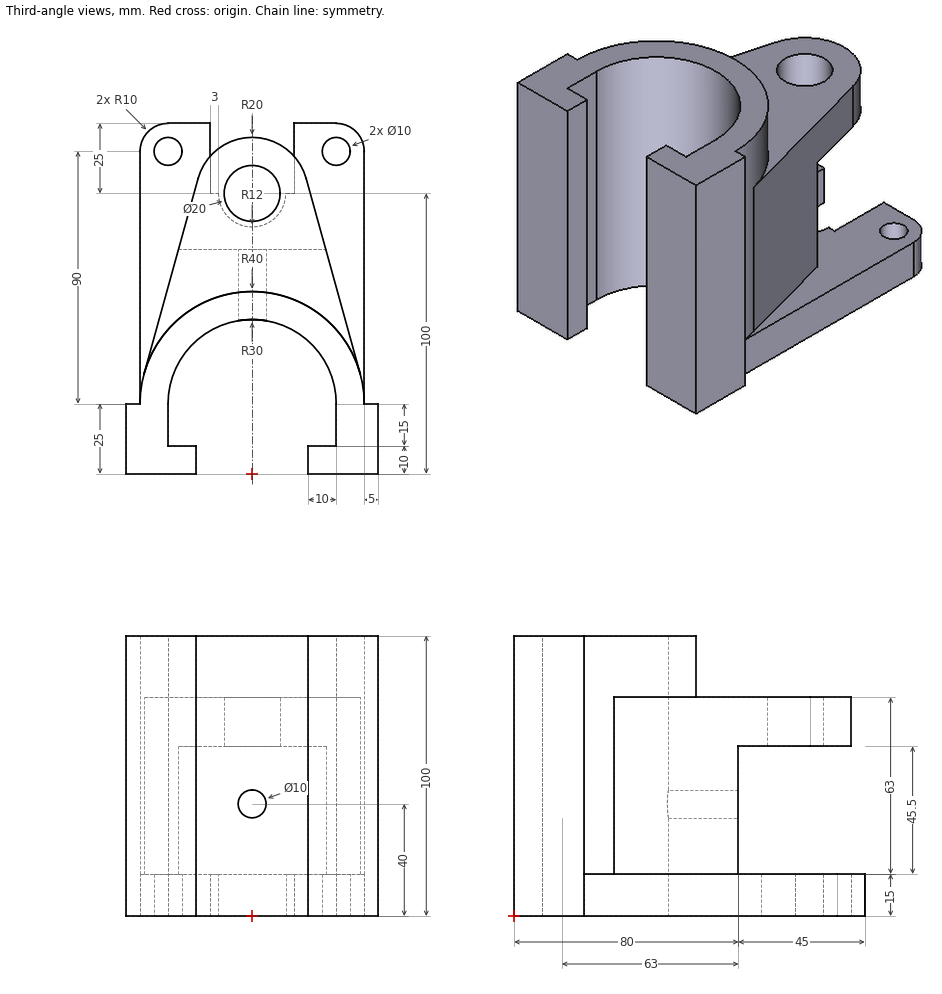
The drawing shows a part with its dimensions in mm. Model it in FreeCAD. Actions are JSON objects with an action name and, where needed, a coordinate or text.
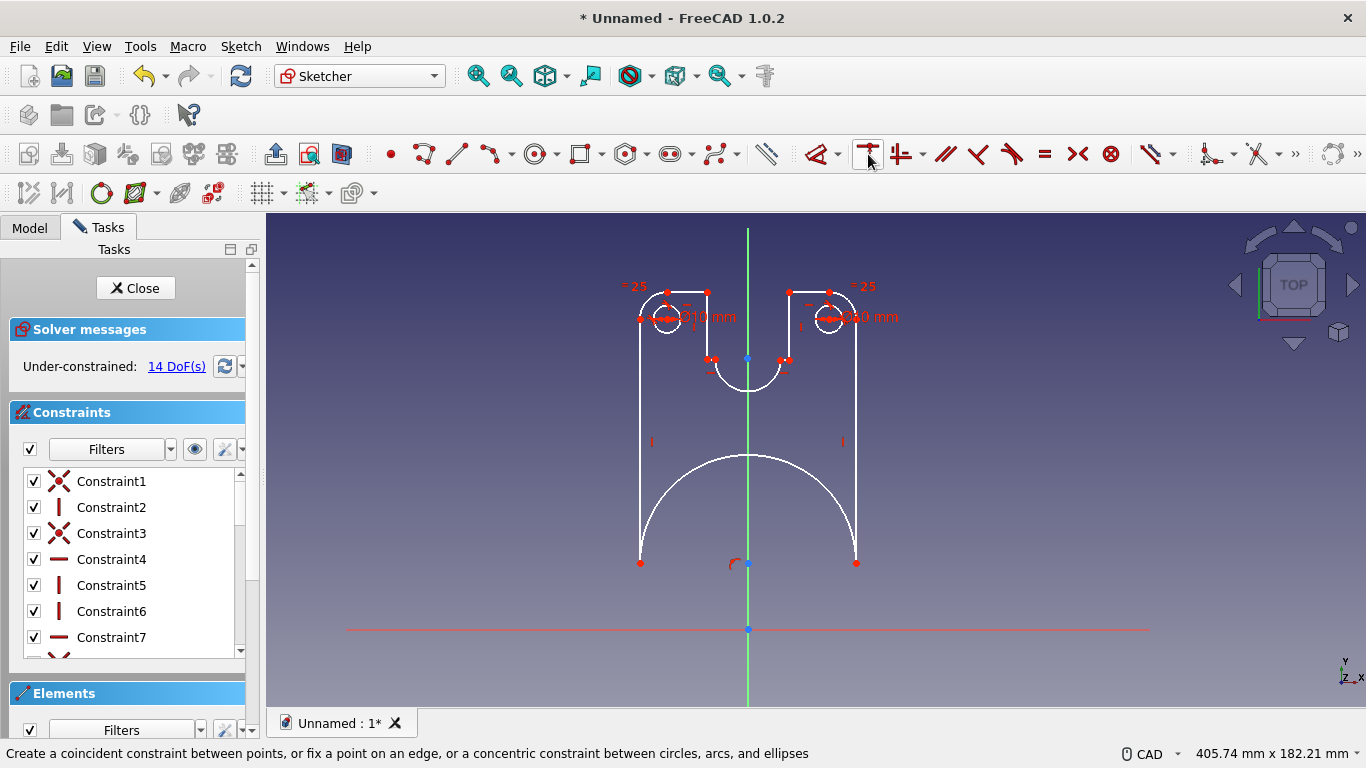
{"action": "left_click", "coordinate": [748, 359]}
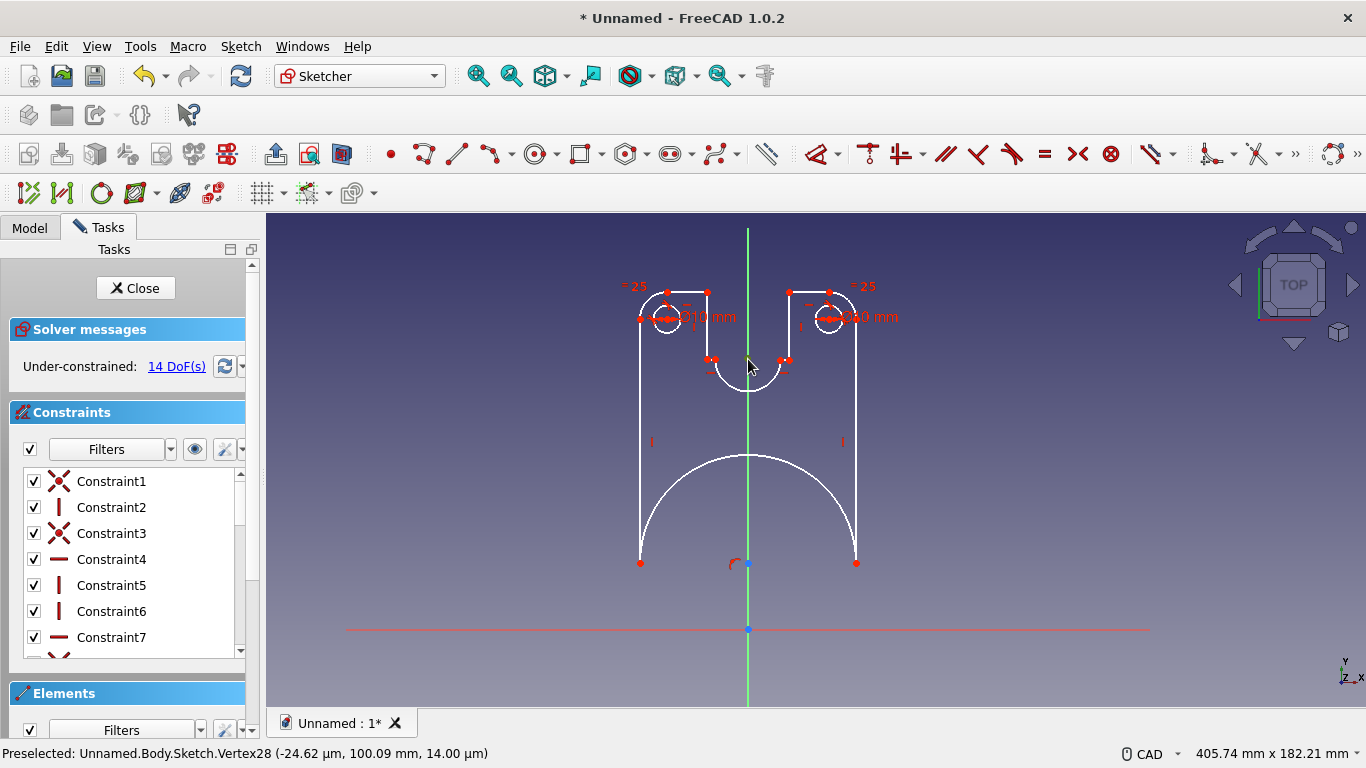
{"action": "left_click", "coordinate": [748, 585]}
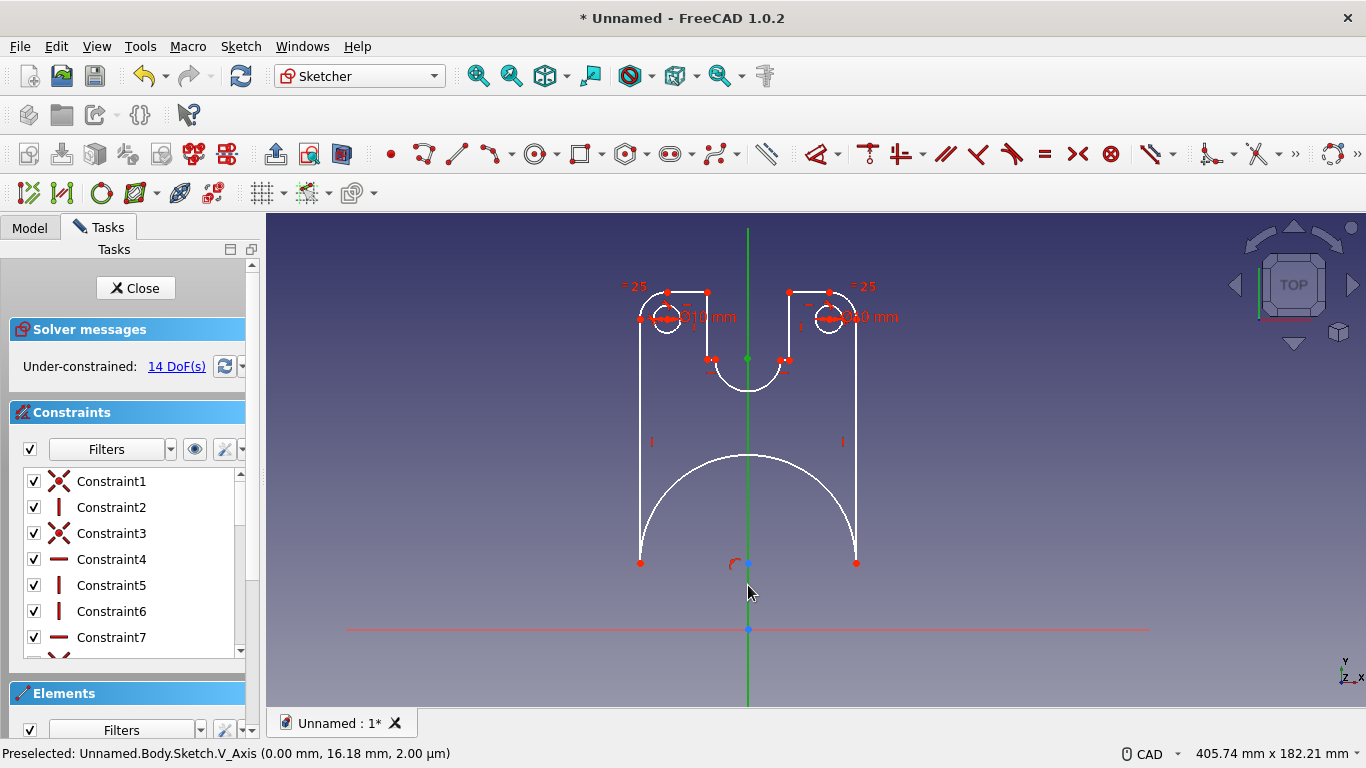
{"action": "left_click", "coordinate": [868, 154]}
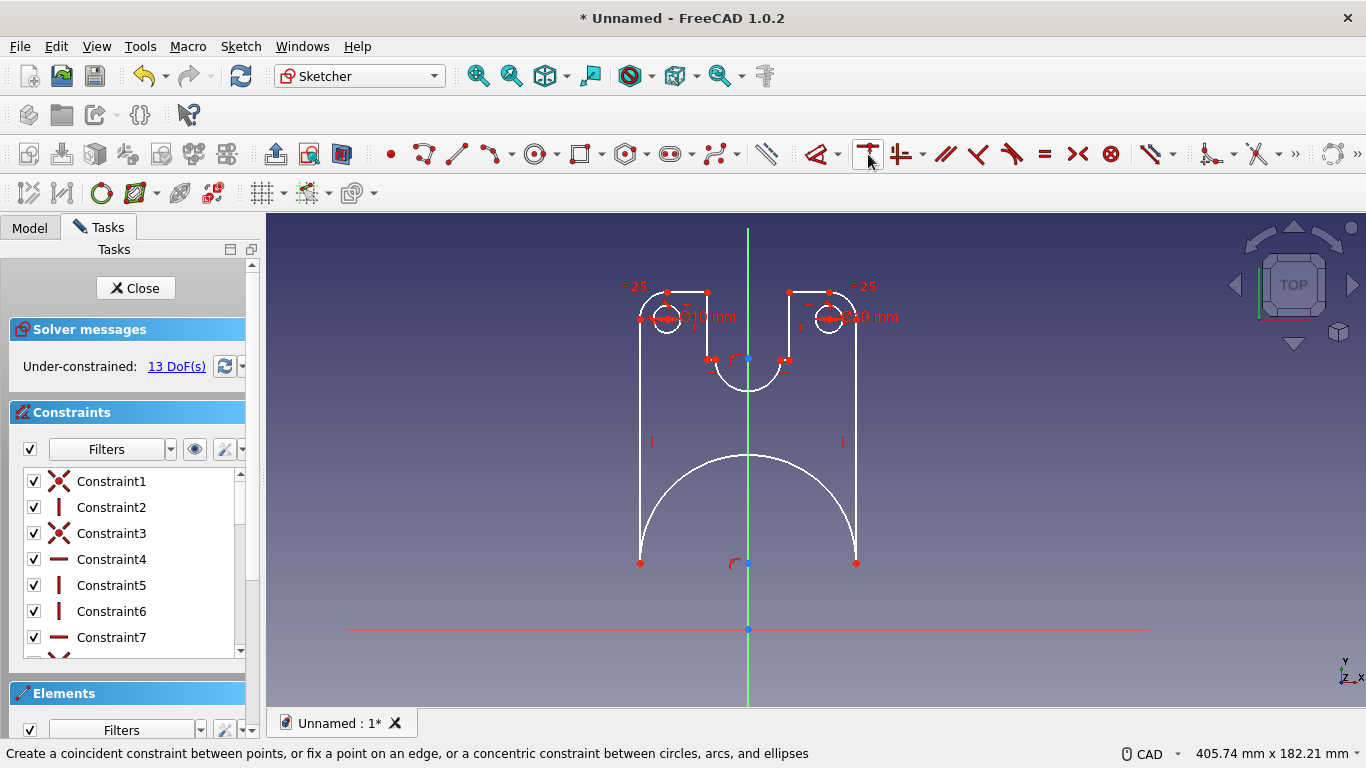
{"action": "left_click", "coordinate": [707, 292]}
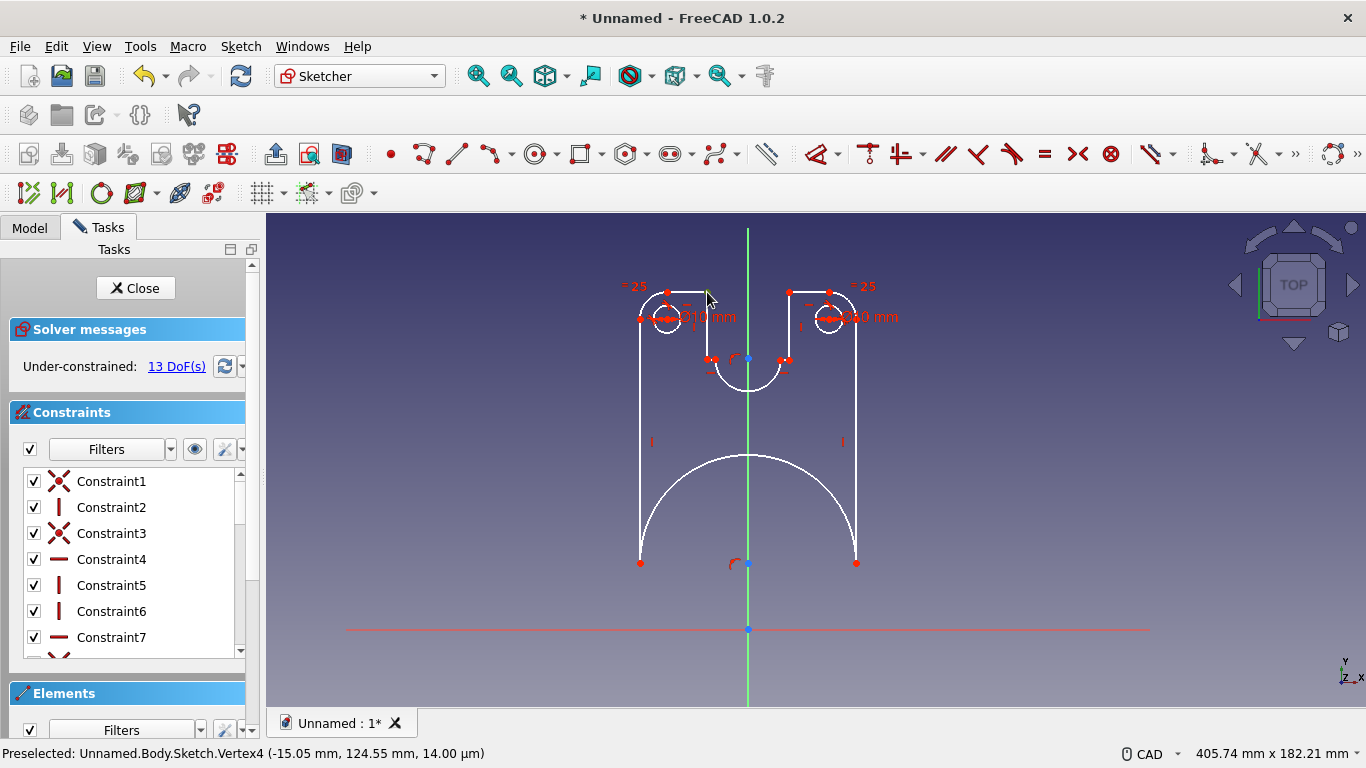
{"action": "left_click", "coordinate": [789, 292]}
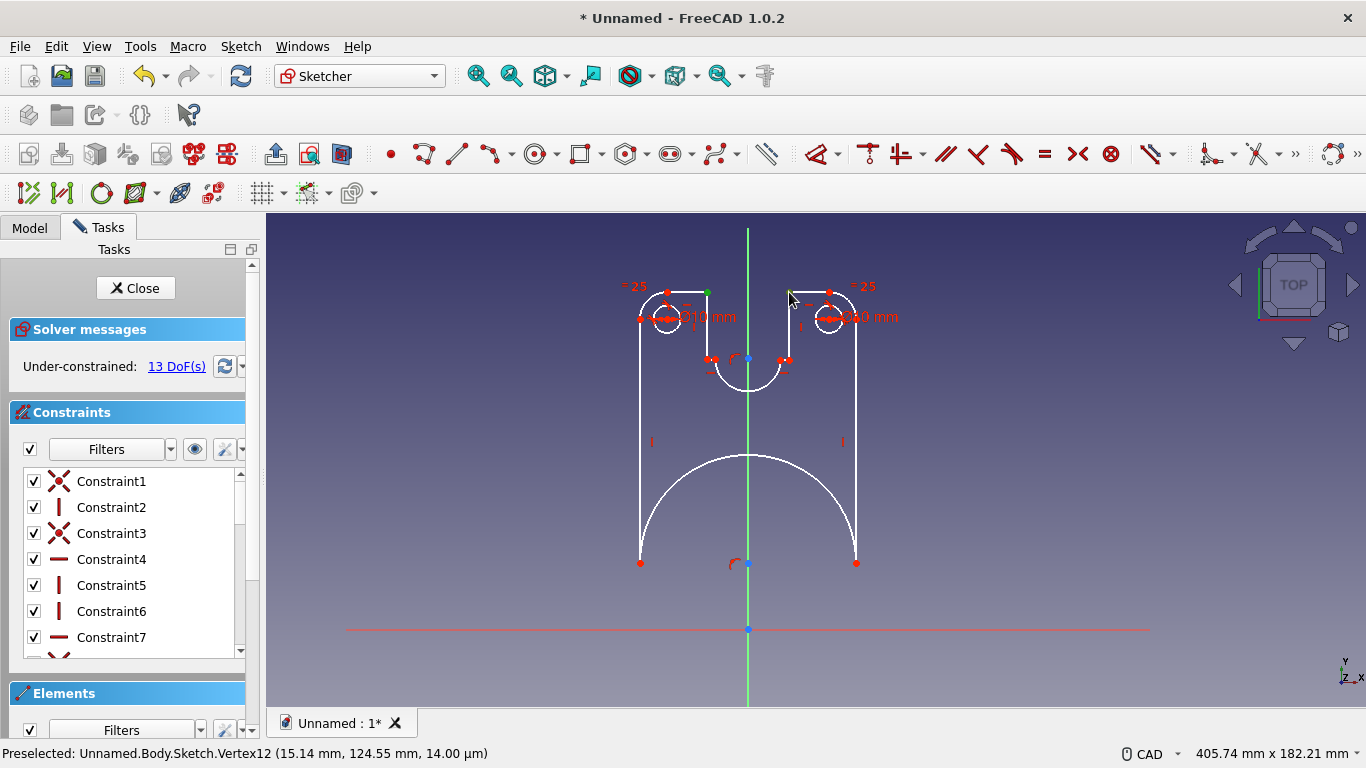
{"action": "left_click", "coordinate": [748, 585]}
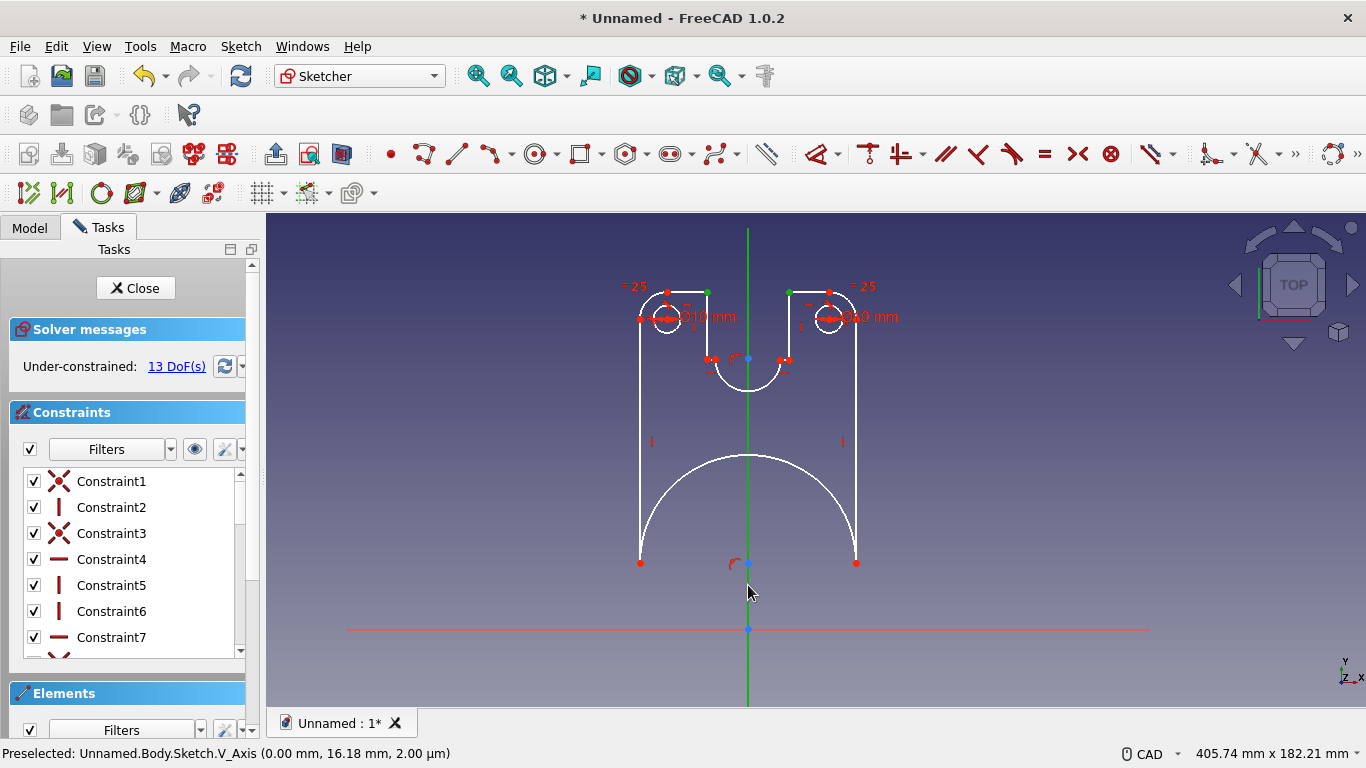
{"action": "left_click", "coordinate": [1078, 154]}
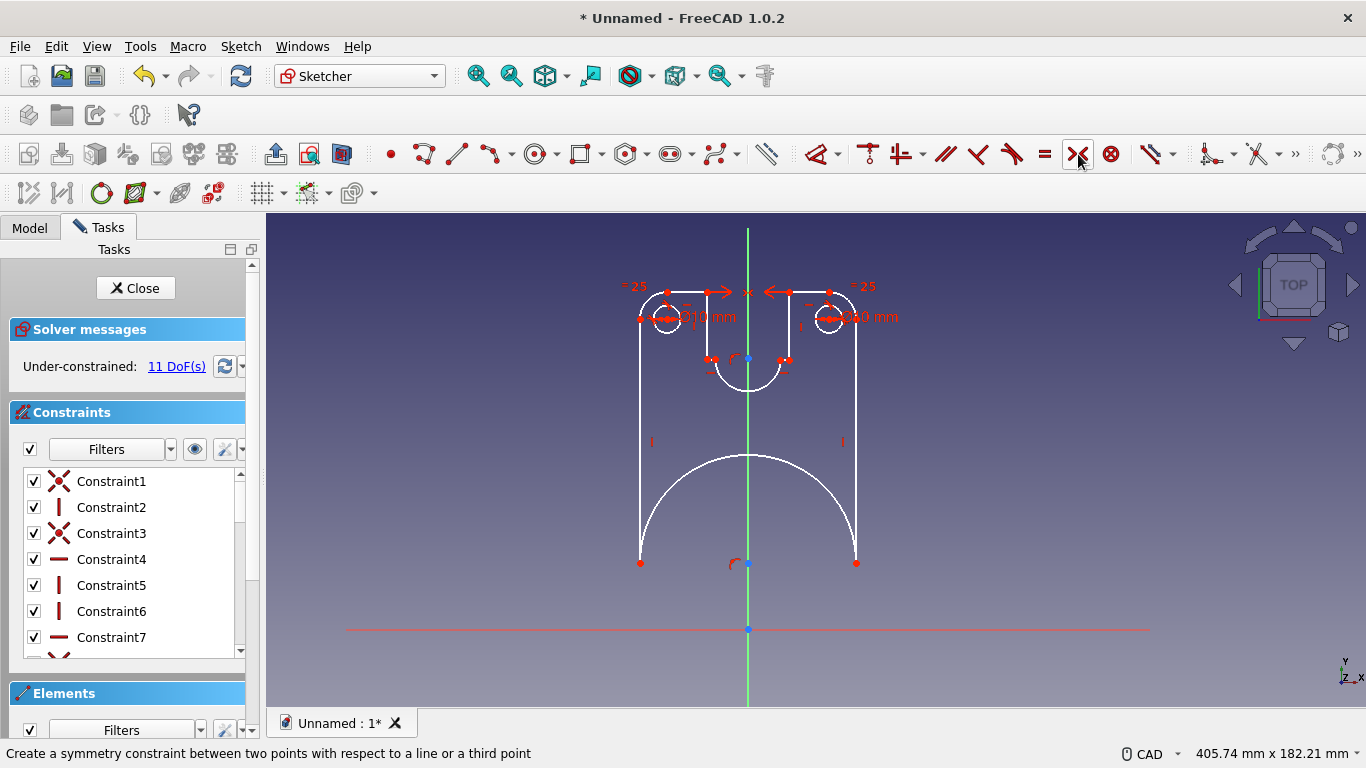
{"action": "left_click", "coordinate": [816, 154]}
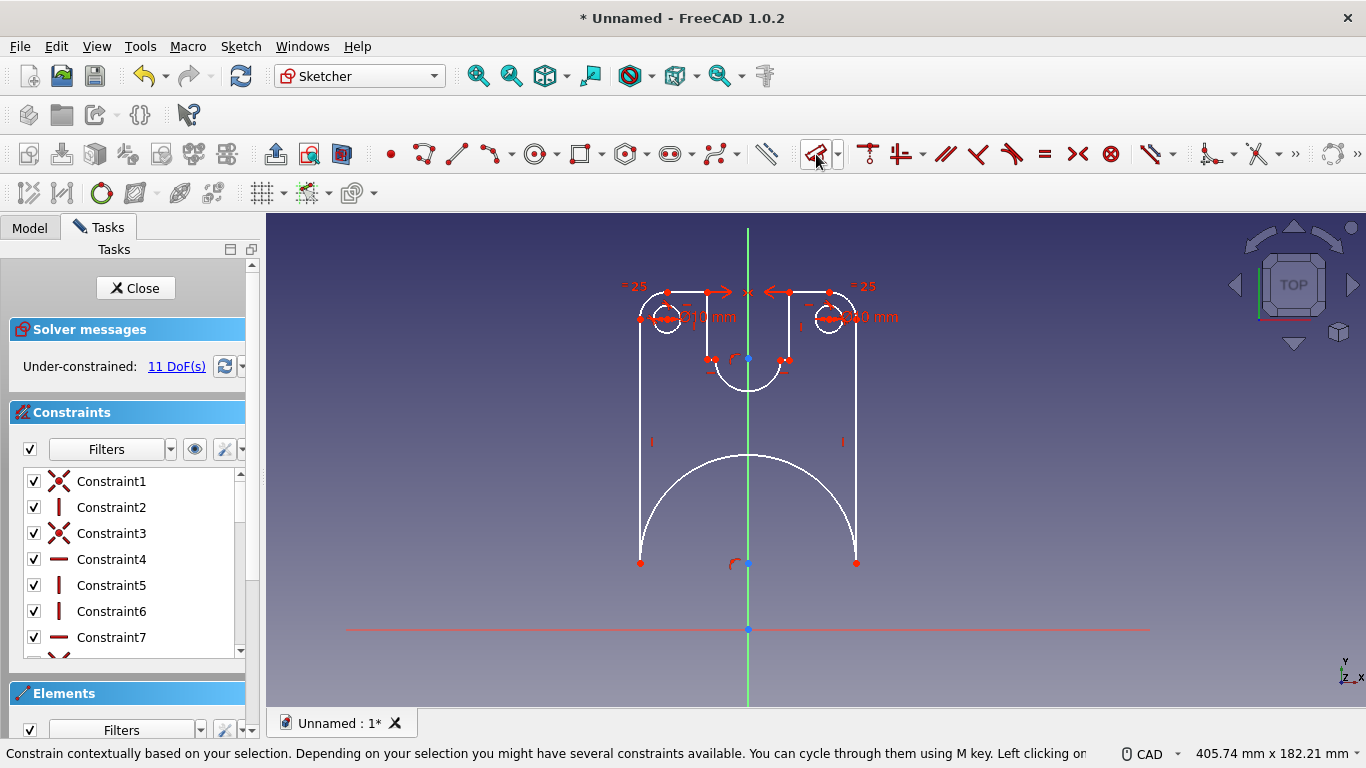
{"action": "scroll", "coordinate": [655, 295], "scroll_direction": "up", "scroll_amount": 2}